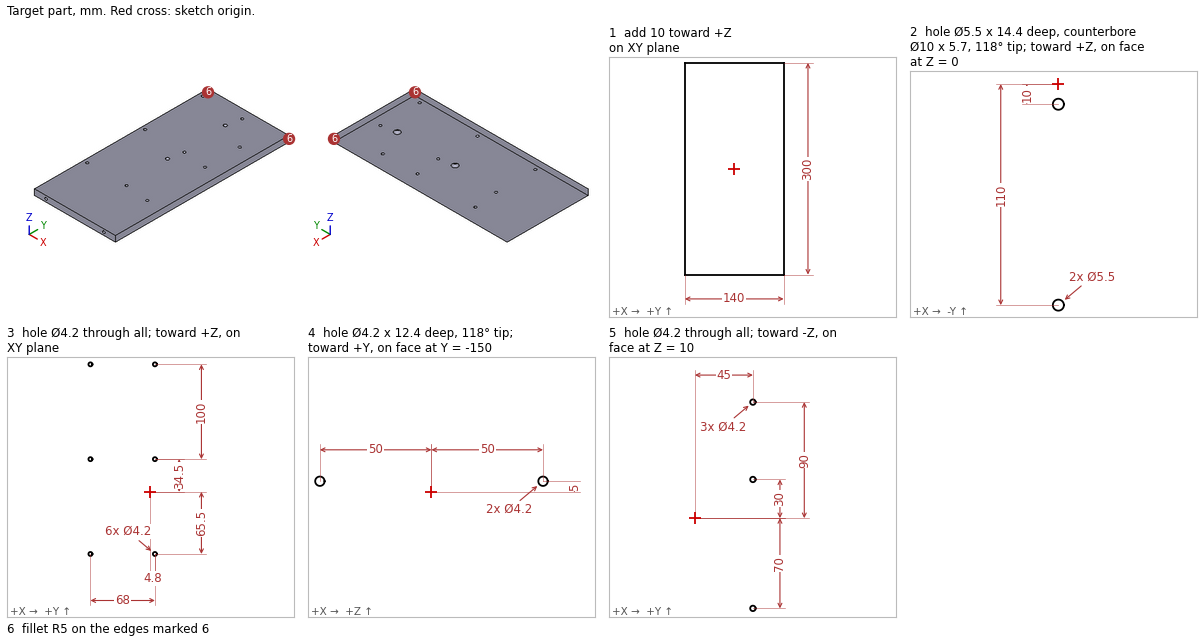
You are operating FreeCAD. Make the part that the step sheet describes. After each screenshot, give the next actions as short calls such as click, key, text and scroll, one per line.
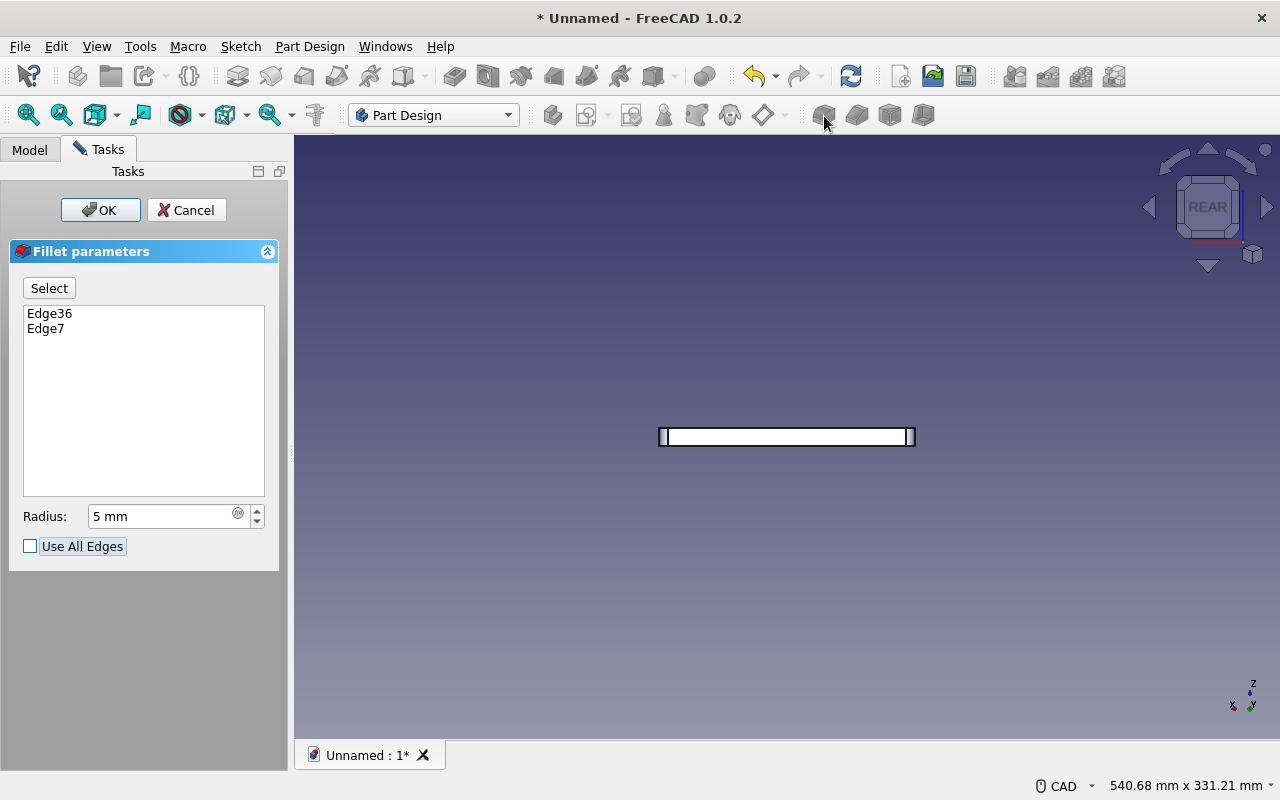
click(101, 210)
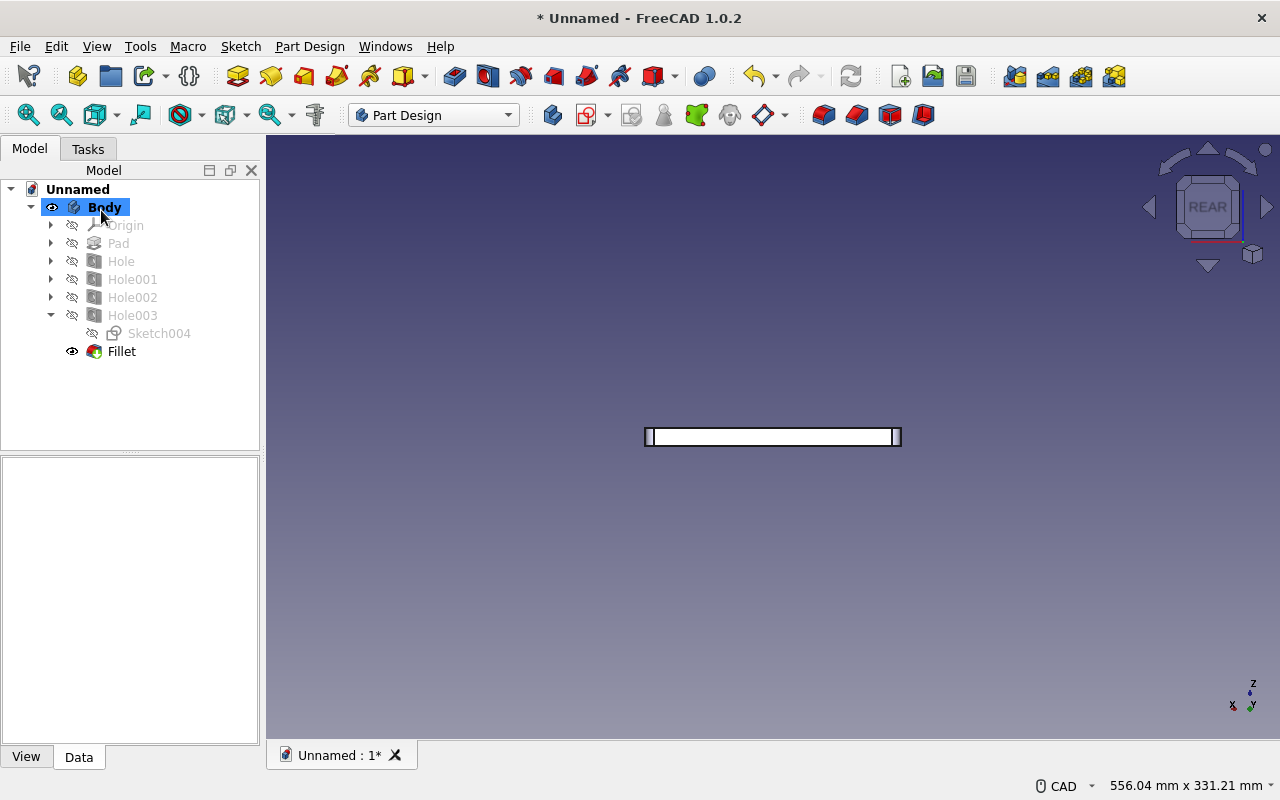
key(0)